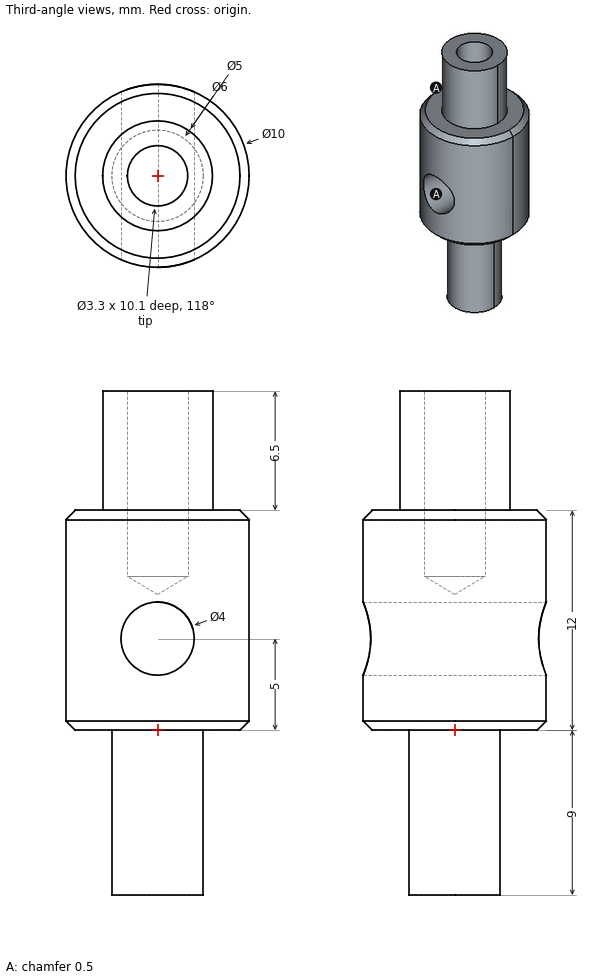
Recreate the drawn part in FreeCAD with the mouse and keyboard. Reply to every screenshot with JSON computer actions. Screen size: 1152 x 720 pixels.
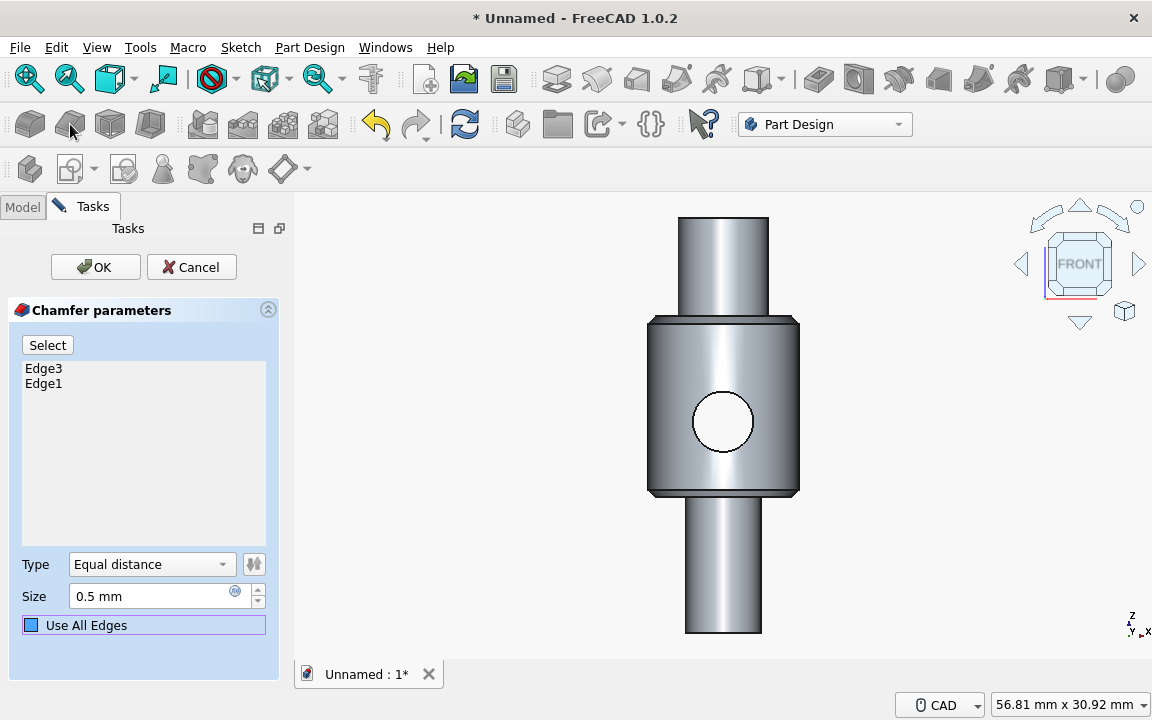
{"action": "left_click", "coordinate": [96, 267]}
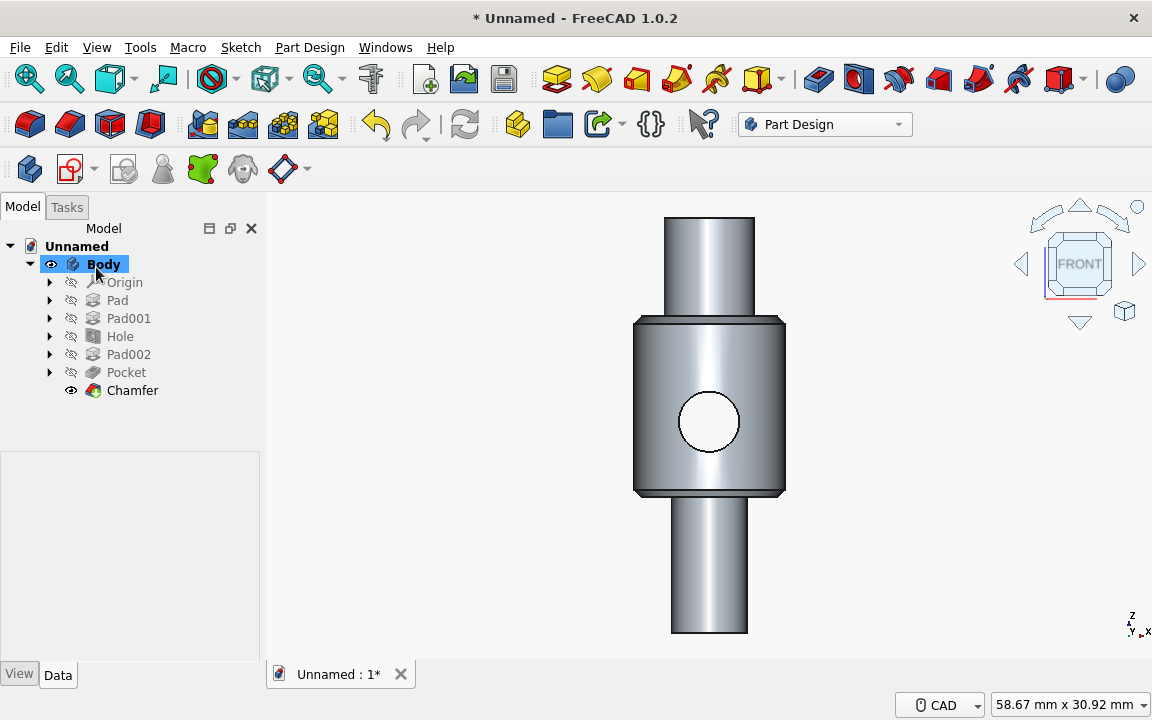
{"action": "key", "text": "0"}